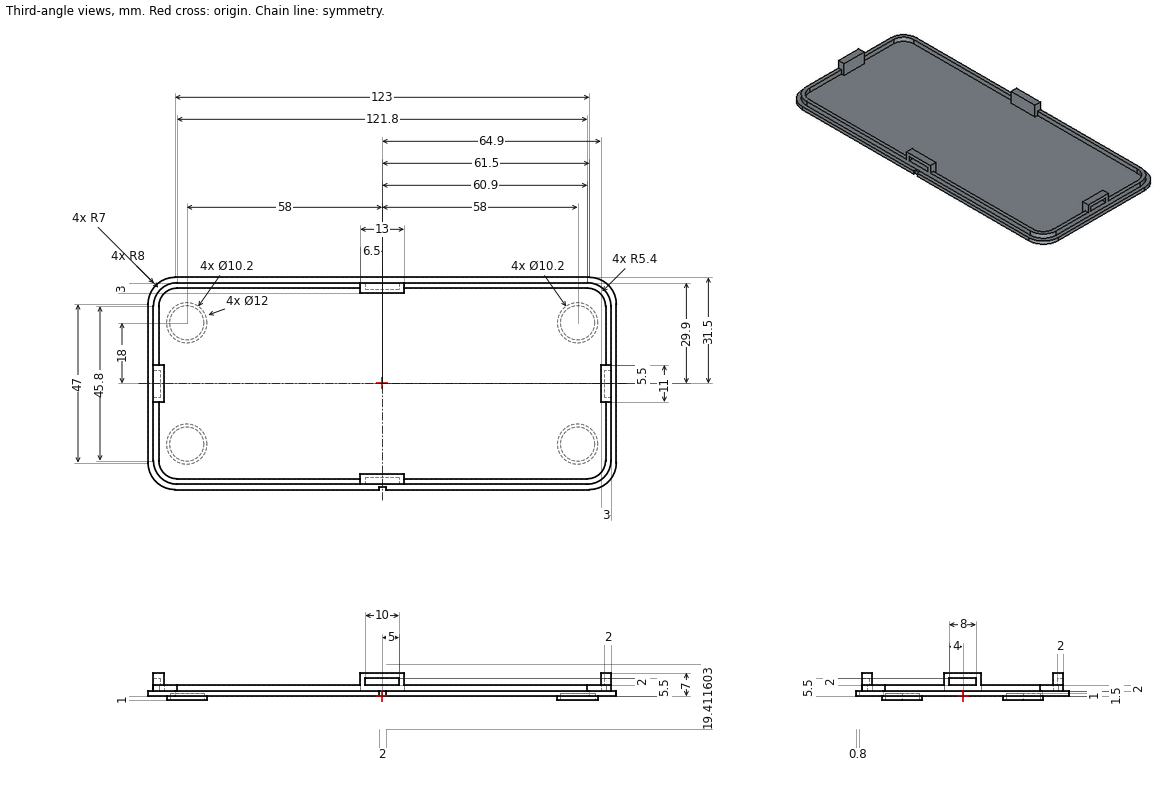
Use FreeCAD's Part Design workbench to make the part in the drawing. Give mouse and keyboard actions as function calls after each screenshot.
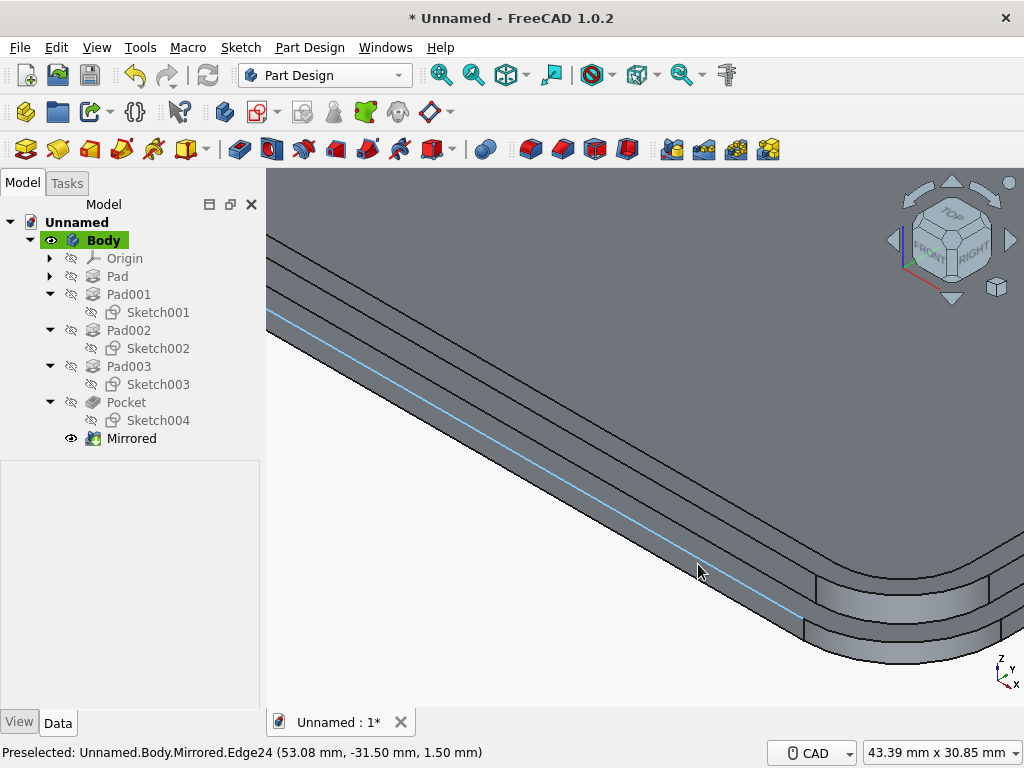
click(695, 566)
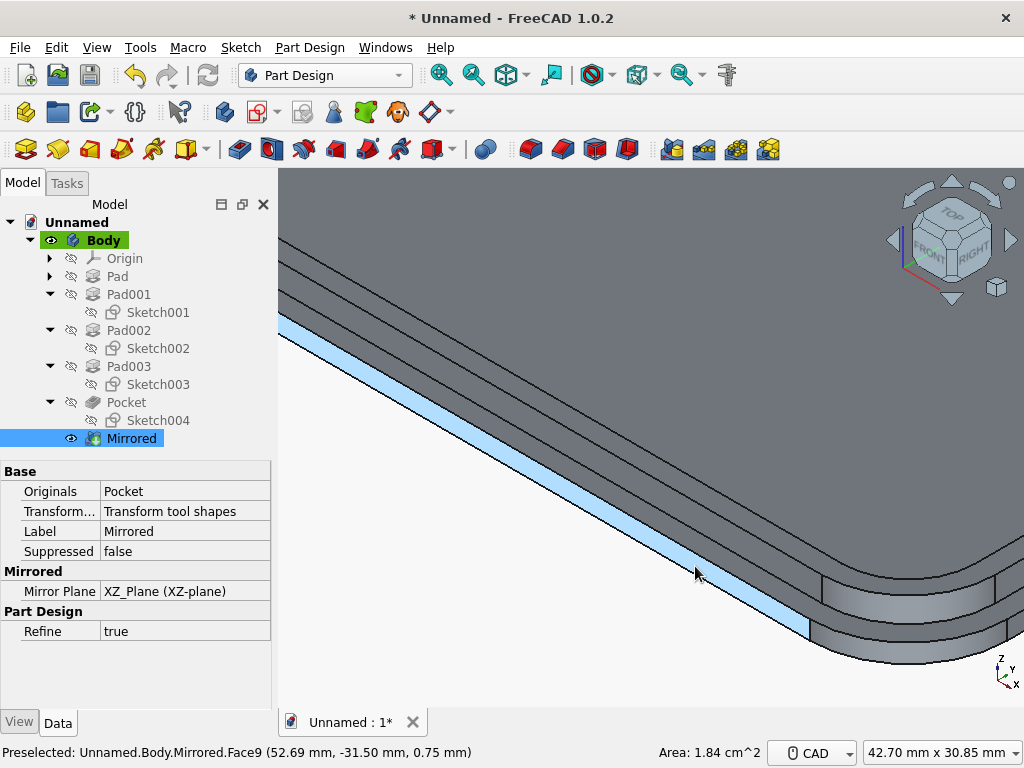
click(258, 112)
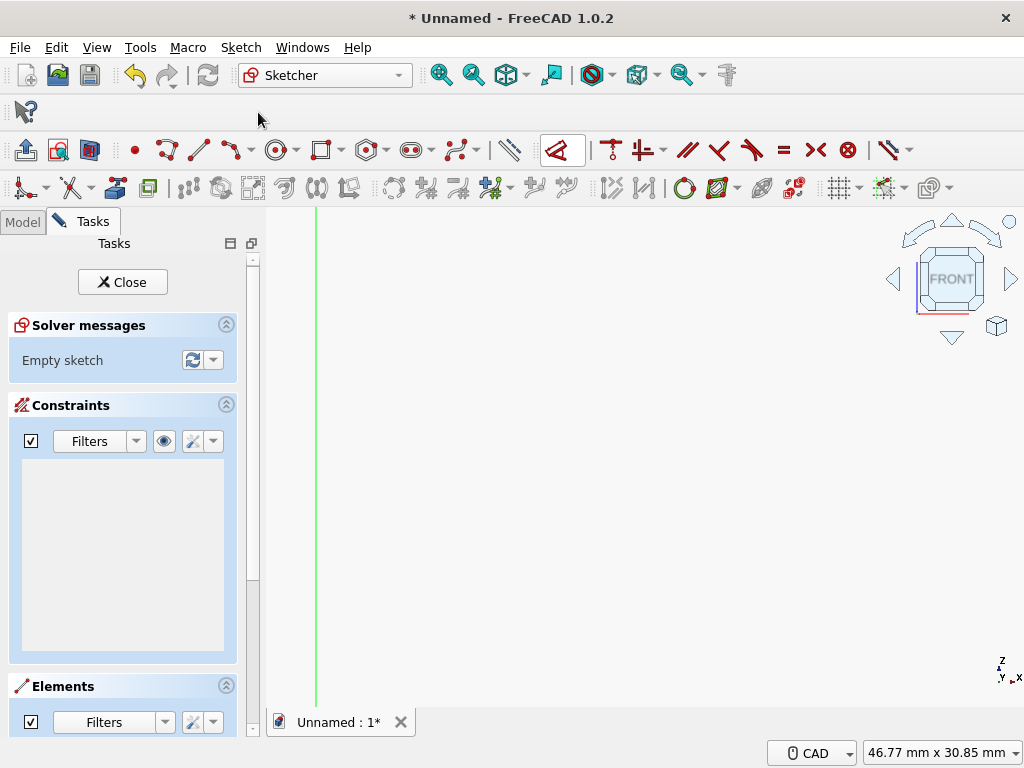
scroll(859, 679, down, 3)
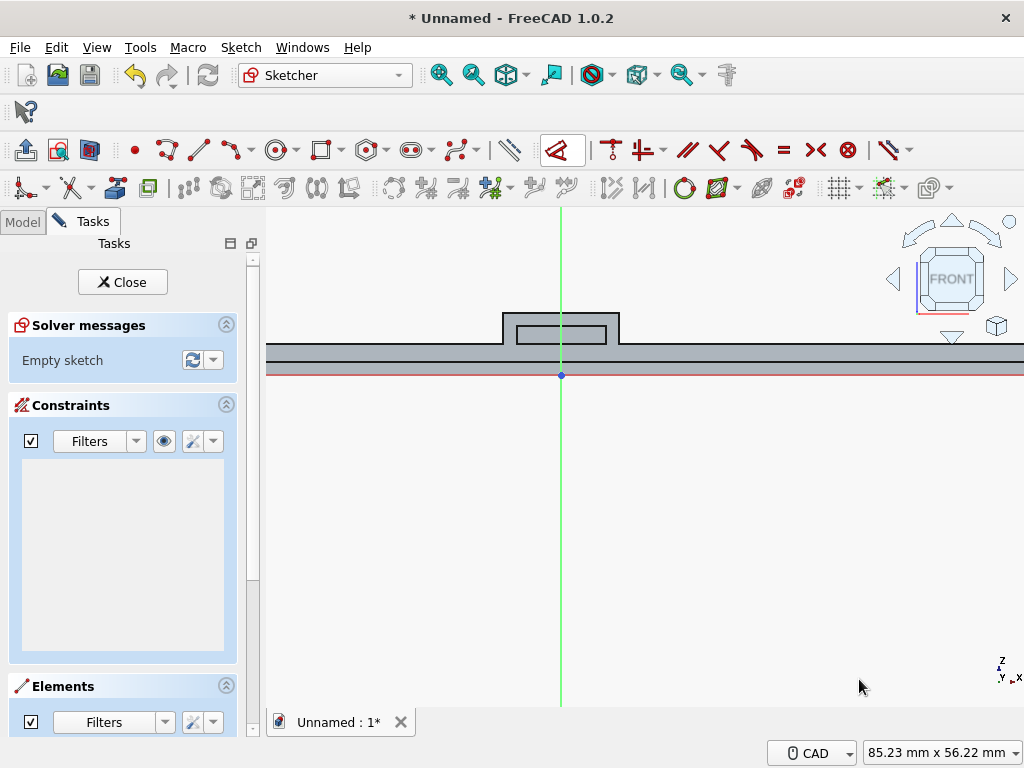
scroll(542, 276, up, 3)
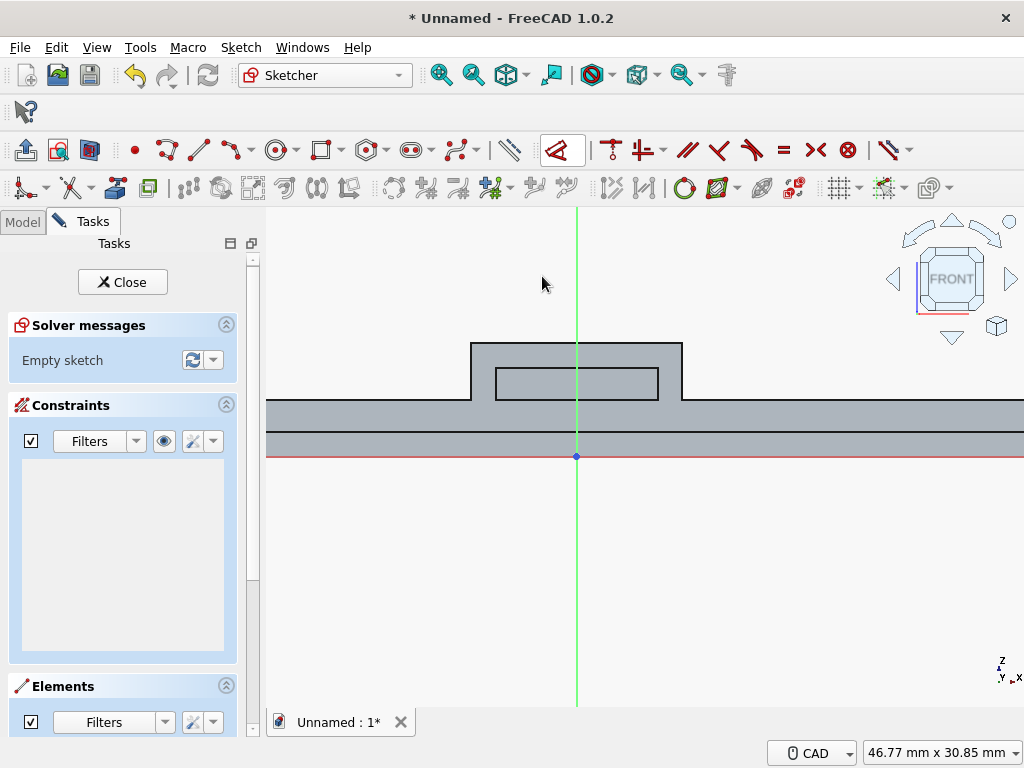
key(g)
key(v)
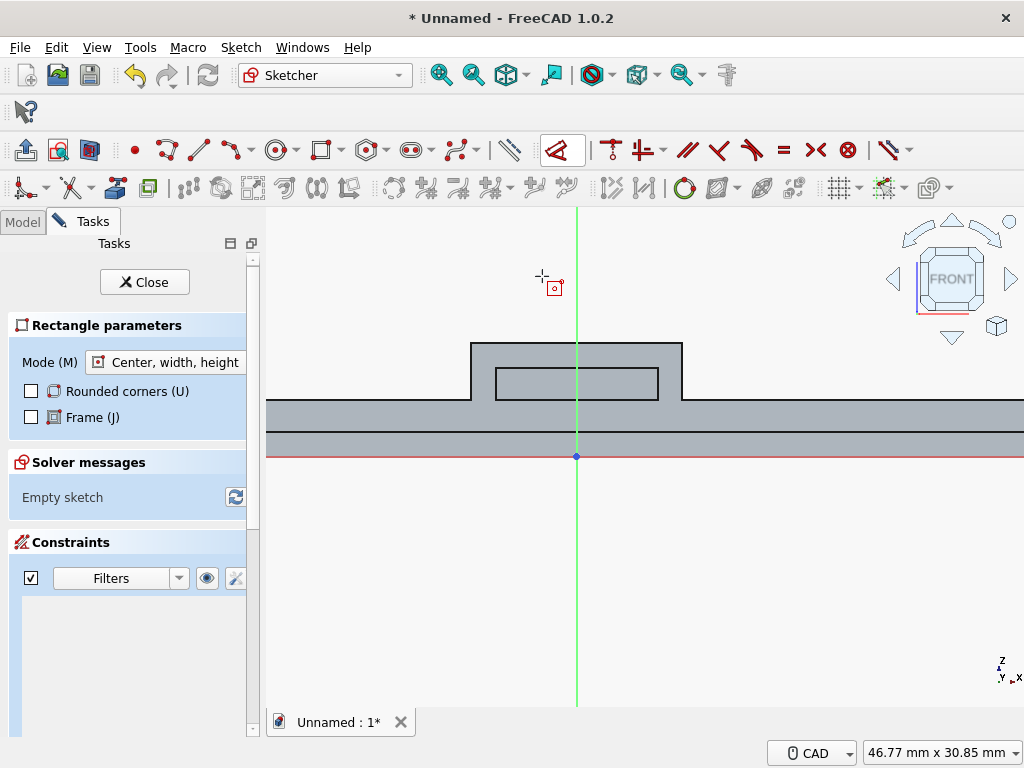
click(577, 457)
click(593, 299)
key(Escape)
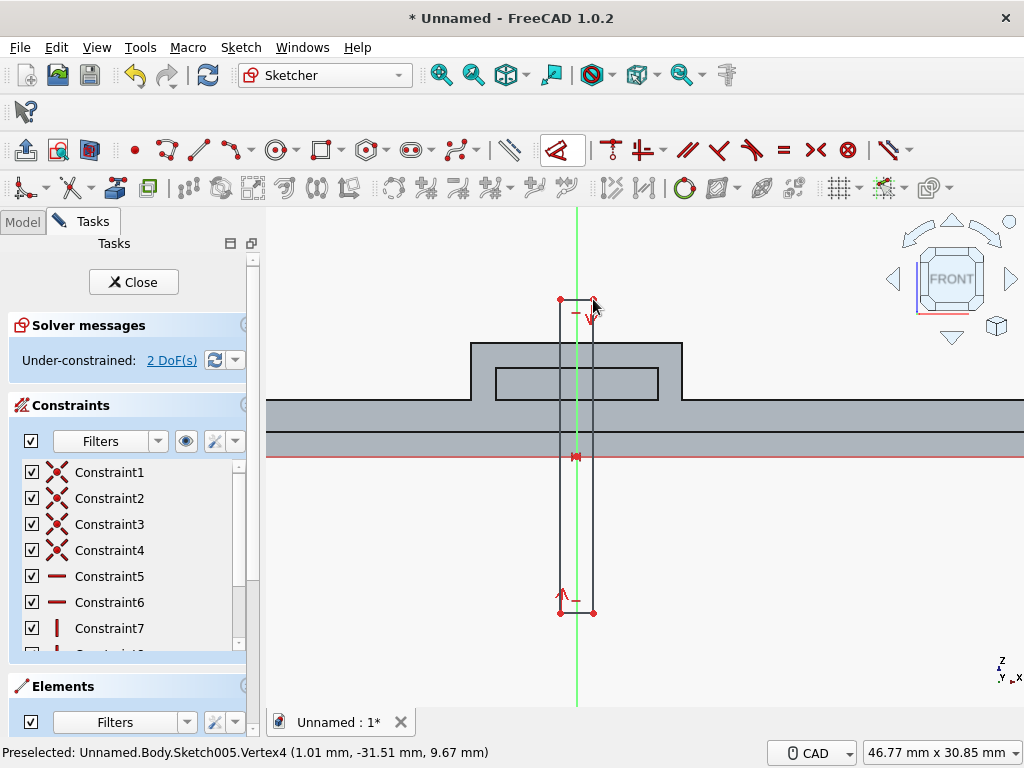
scroll(573, 613, up, 2)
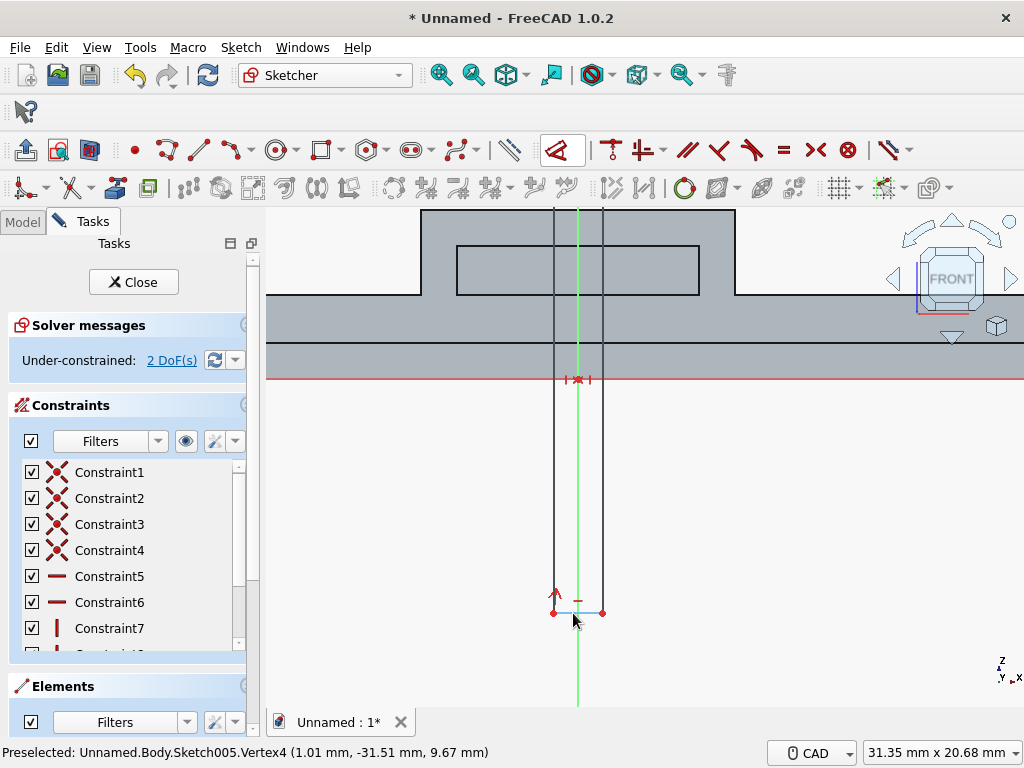
click(573, 613)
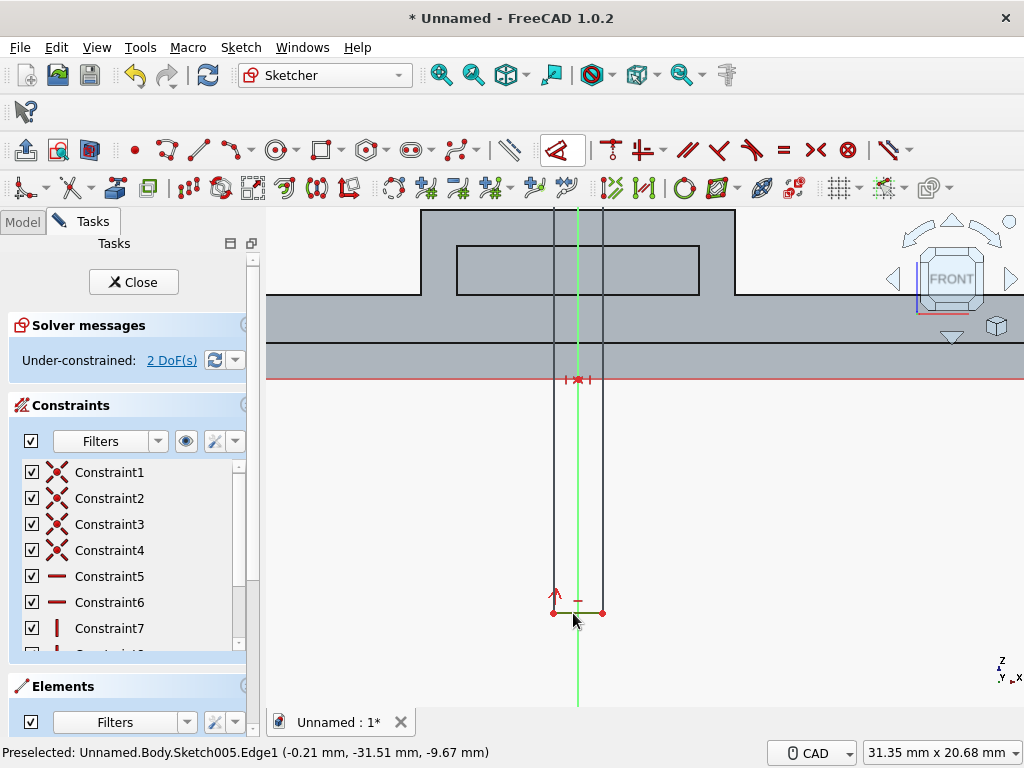
key(l)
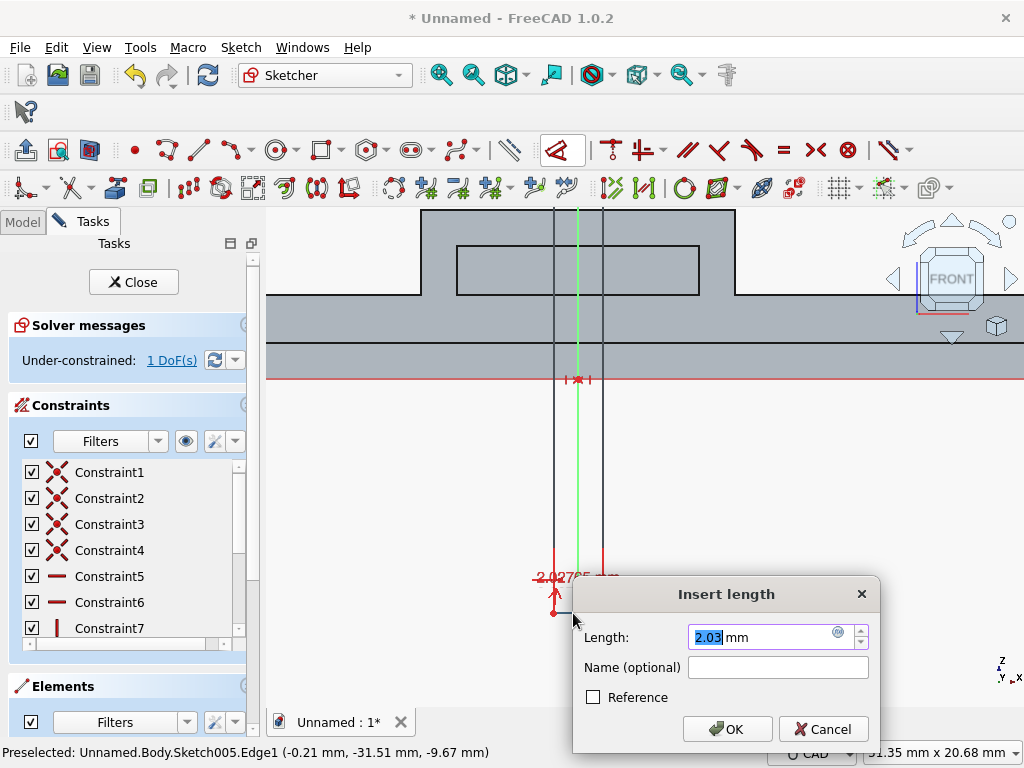
text(2)
key(Return)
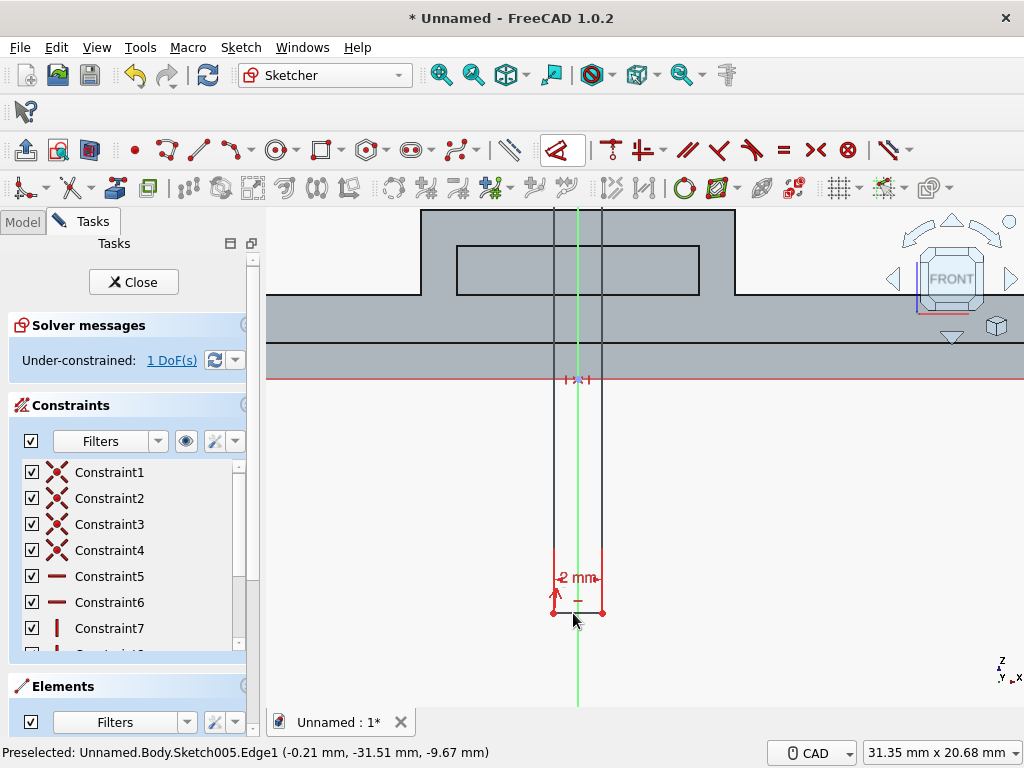
click(602, 473)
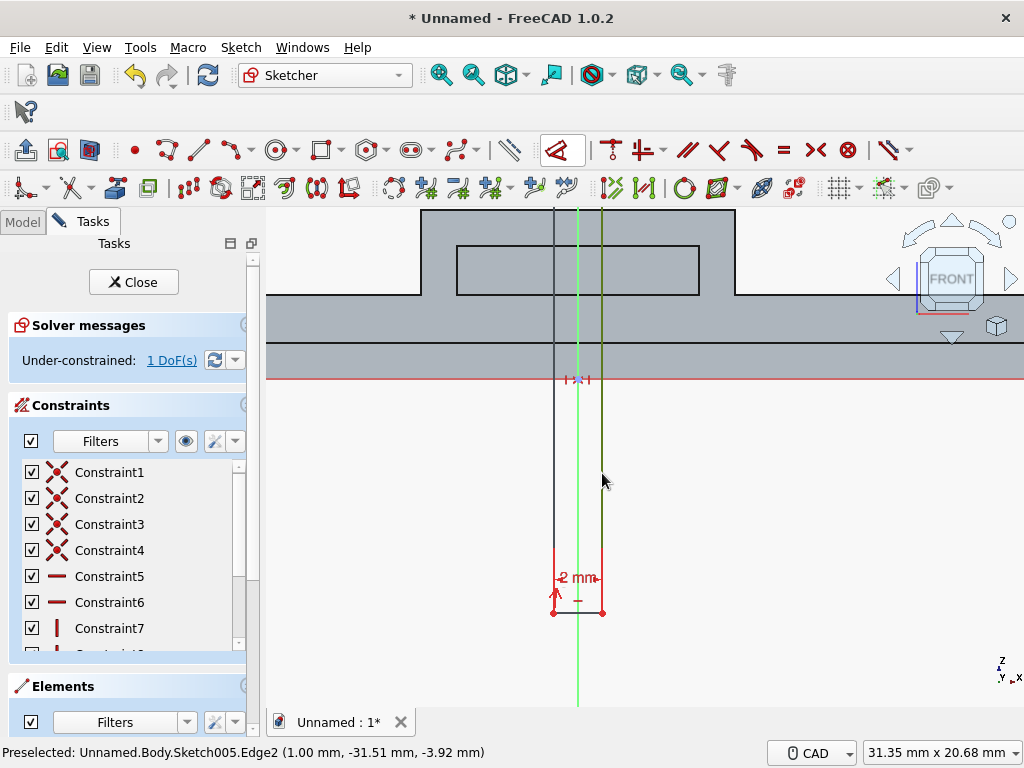
key(i)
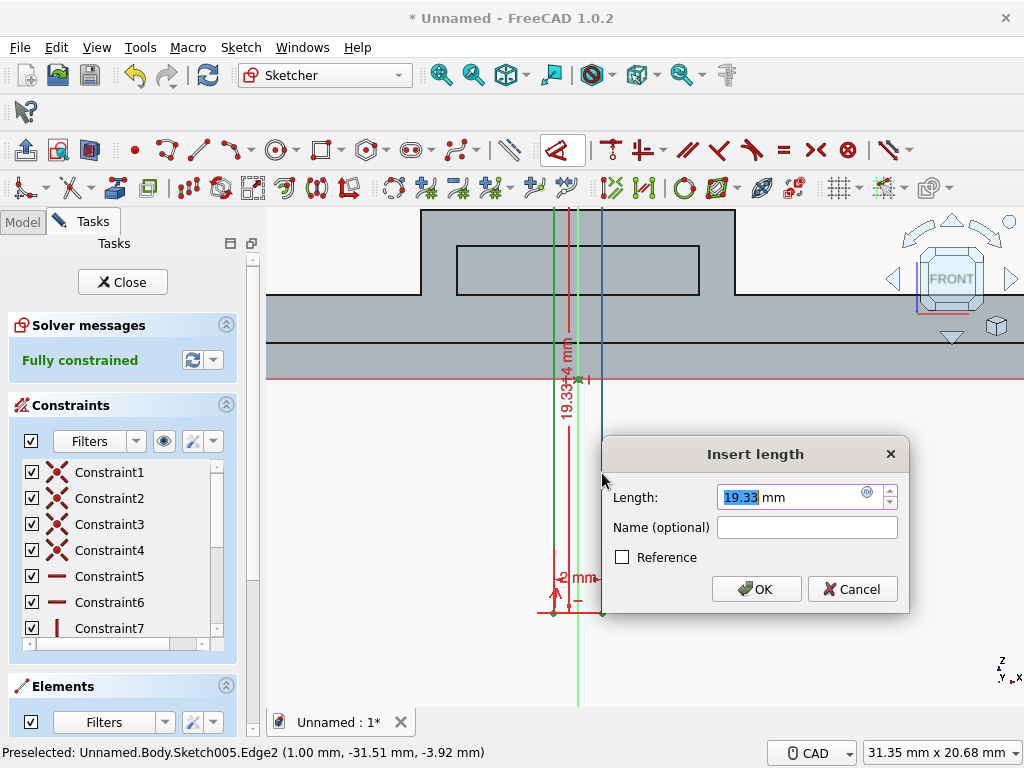
text(19.411603)
key(Return)